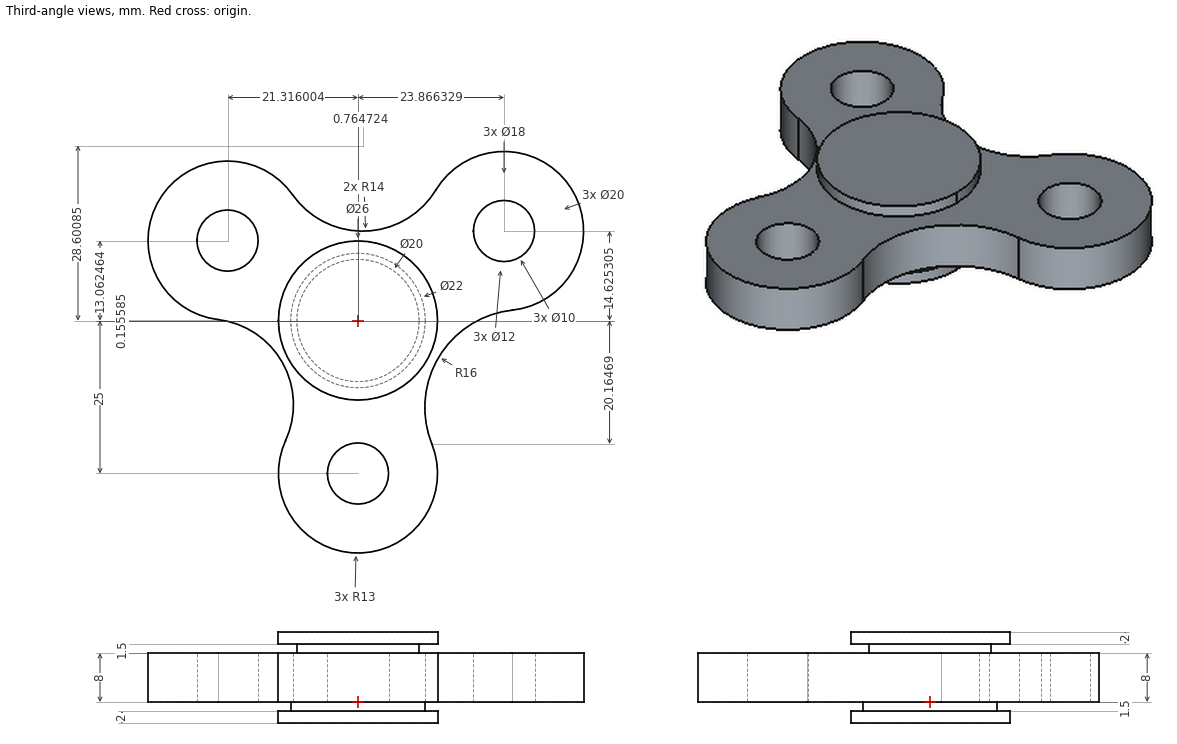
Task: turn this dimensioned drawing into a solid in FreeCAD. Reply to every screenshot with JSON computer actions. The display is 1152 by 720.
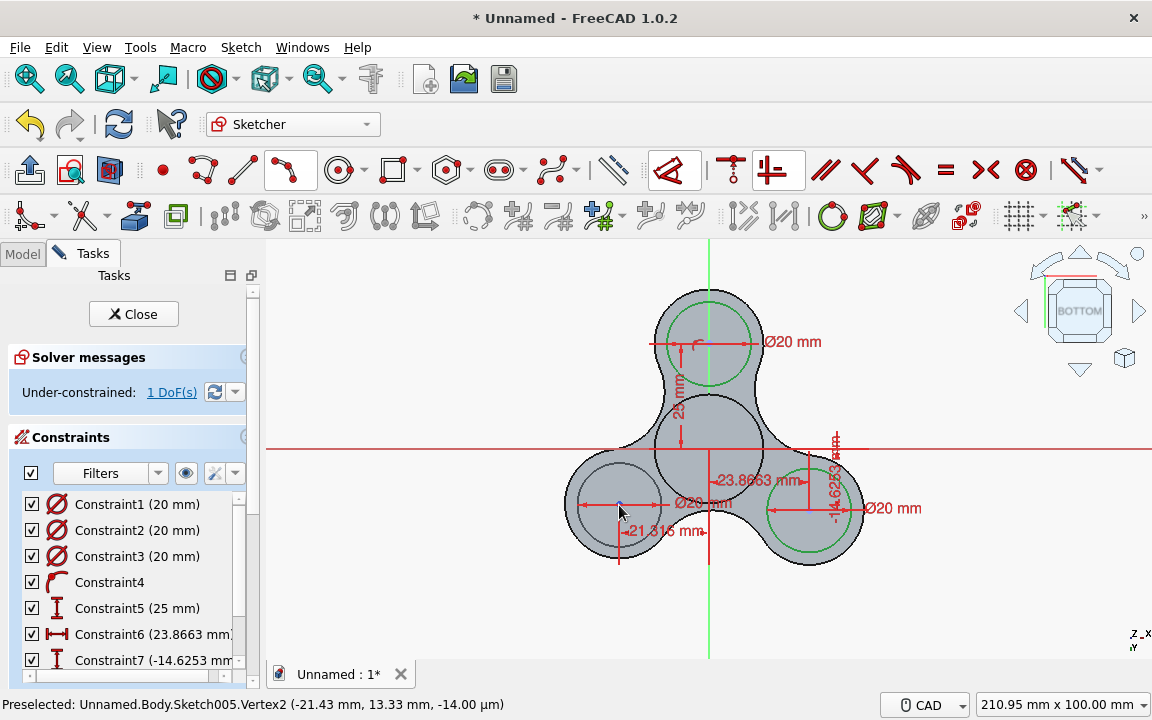
{"action": "left_click", "coordinate": [619, 505]}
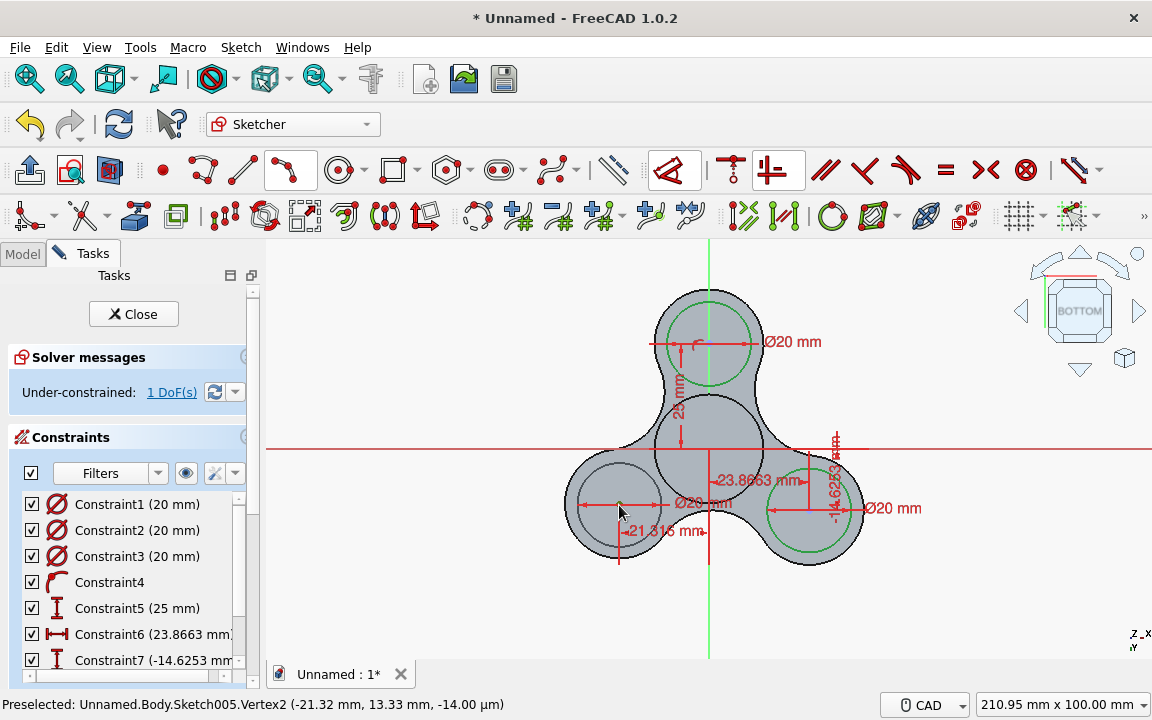
{"action": "key", "text": "i"}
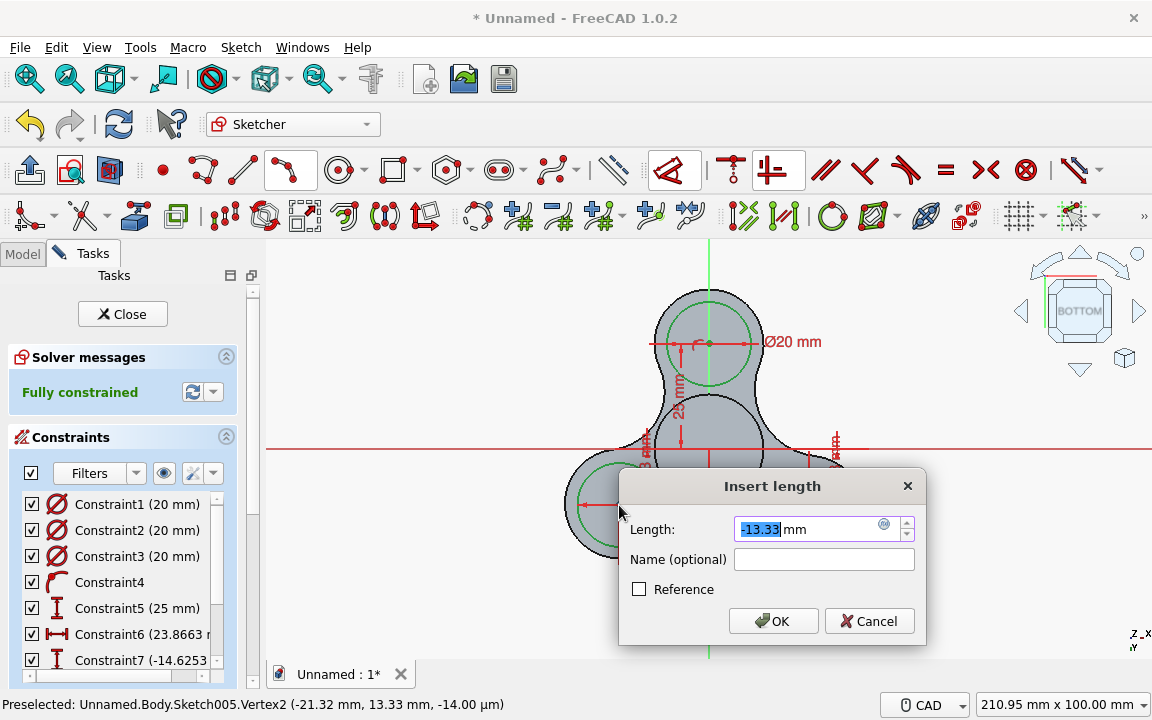
{"action": "type", "text": "-13.062464"}
{"action": "key", "text": "Return"}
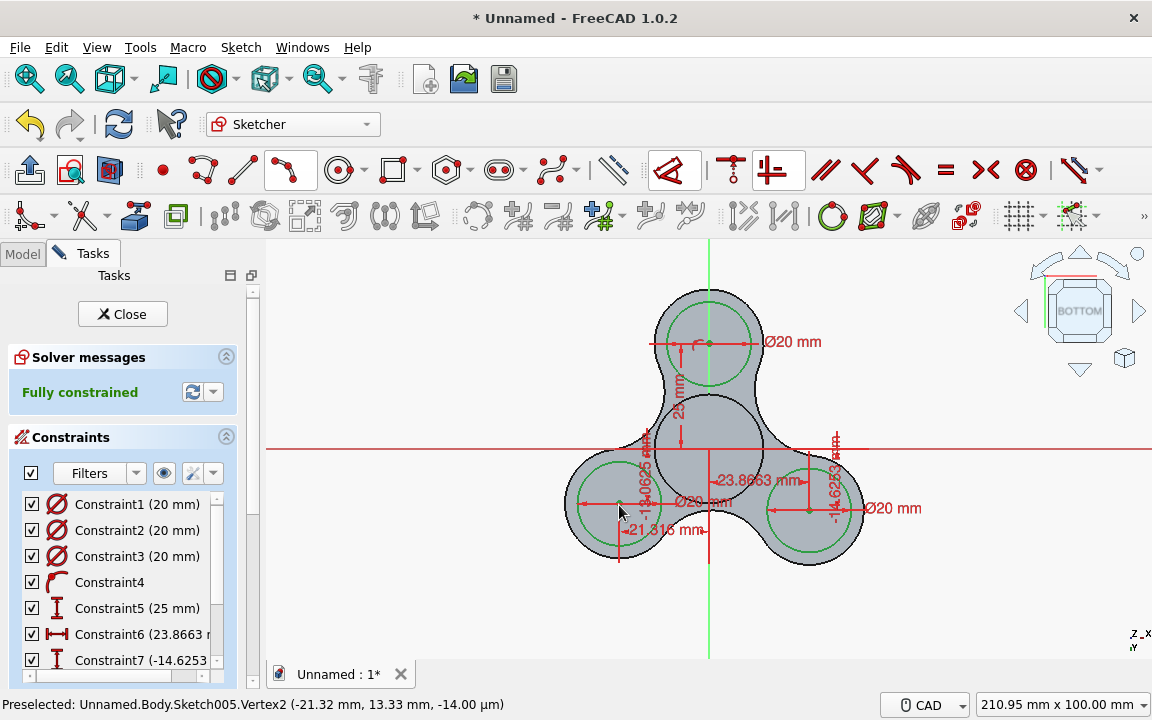
{"action": "left_click", "coordinate": [123, 314]}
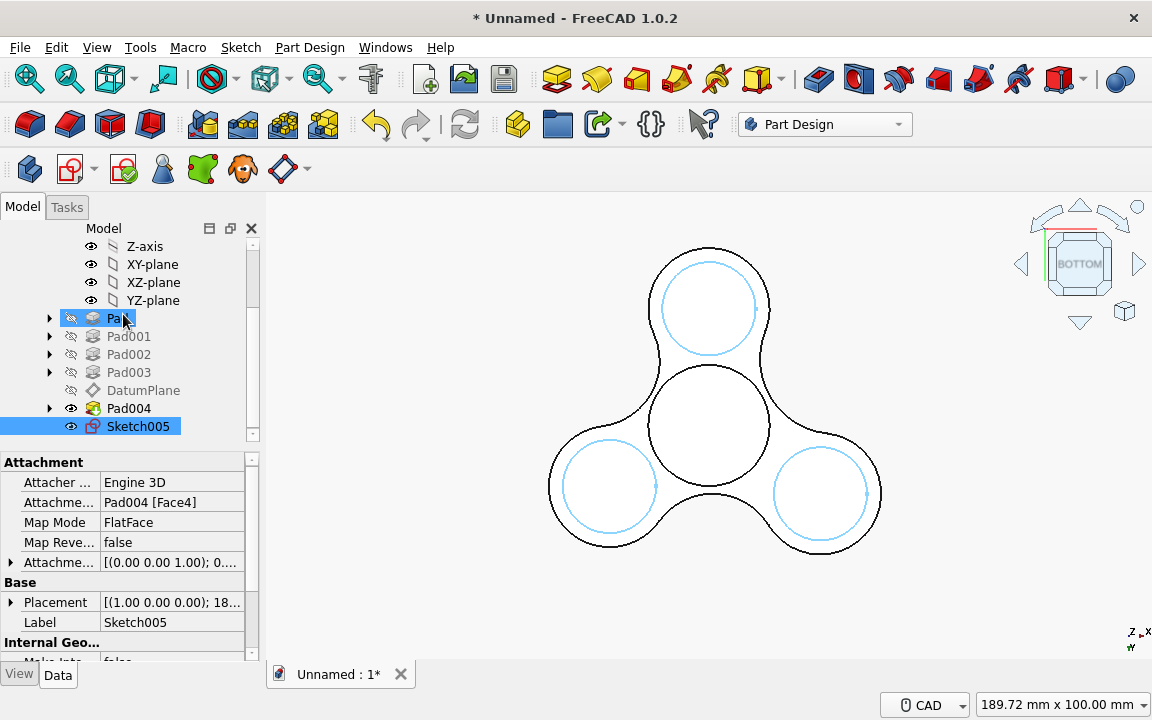
{"action": "left_click", "coordinate": [820, 80]}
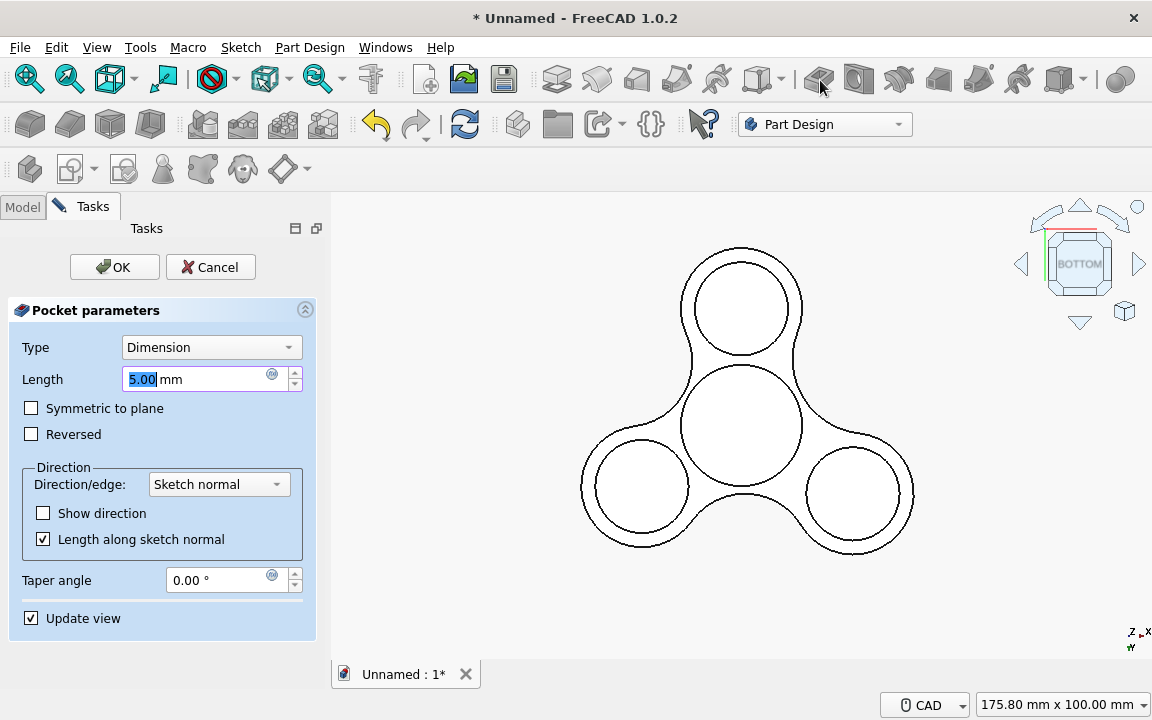
{"action": "type", "text": "8"}
{"action": "key", "text": "Tab"}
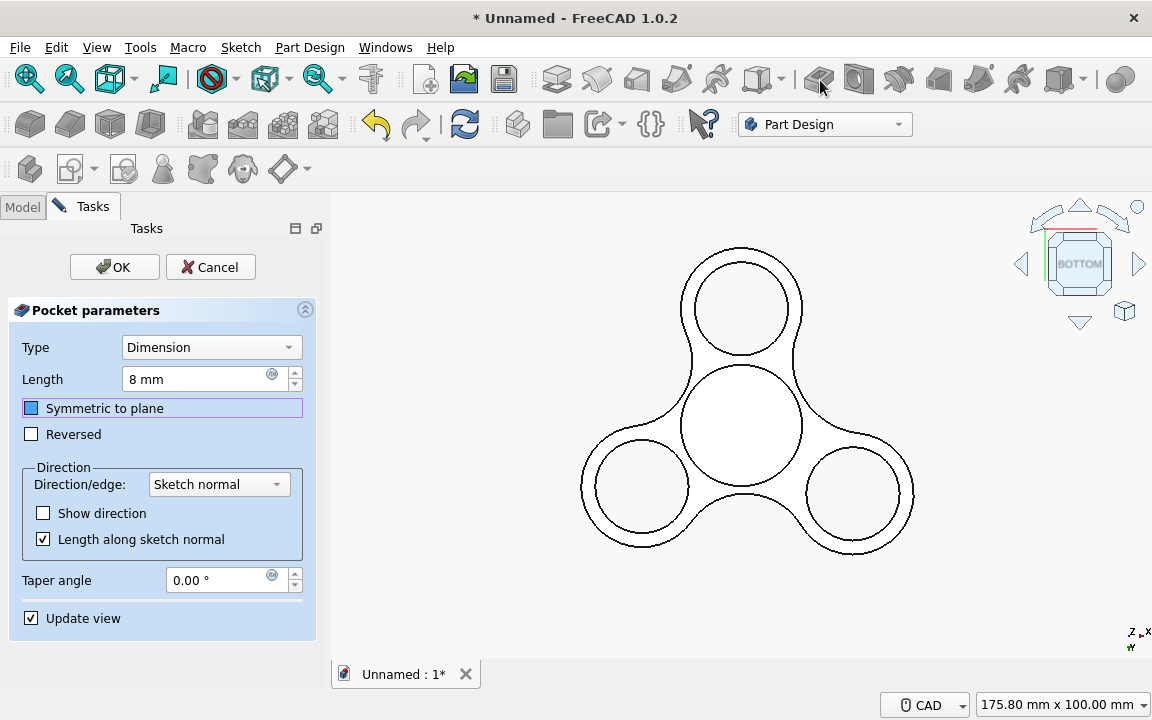
{"action": "left_click", "coordinate": [115, 267]}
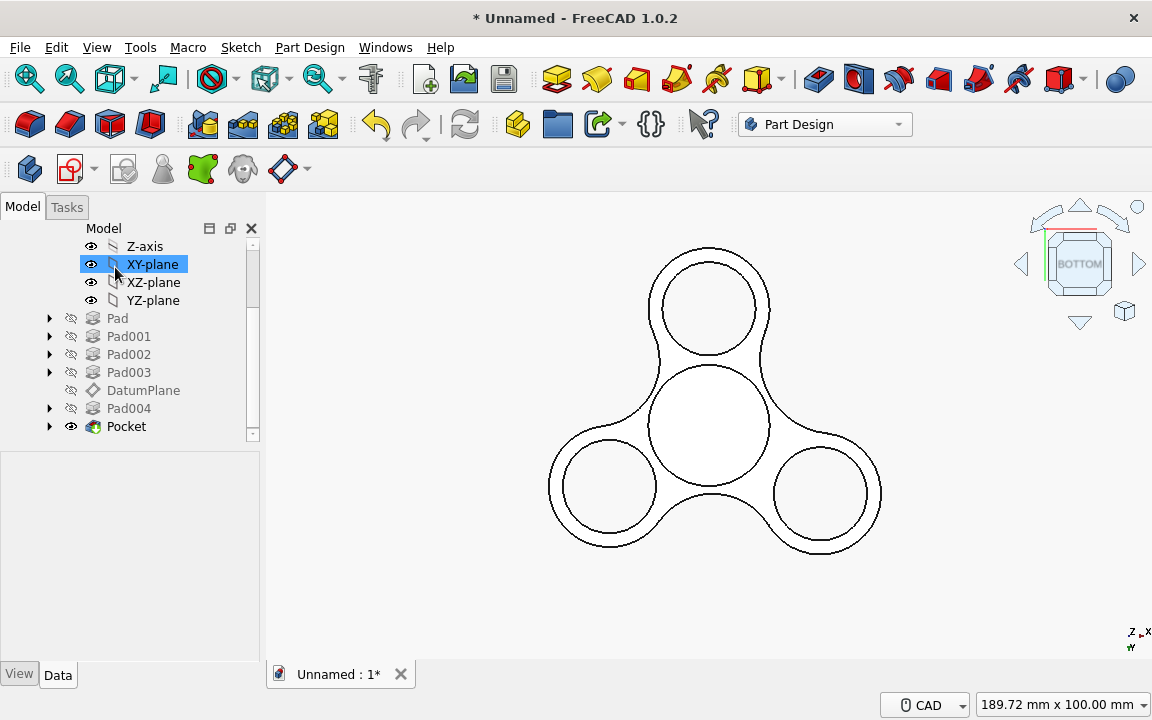
{"action": "left_click", "coordinate": [762, 488]}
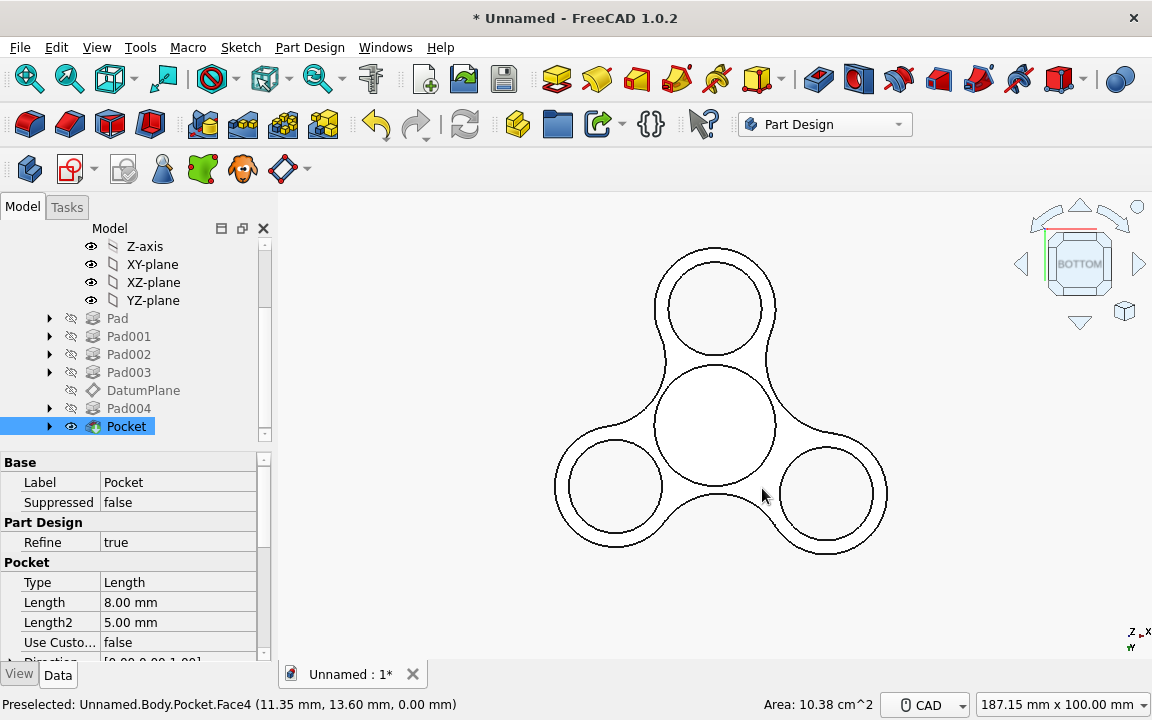
{"action": "left_click", "coordinate": [70, 170]}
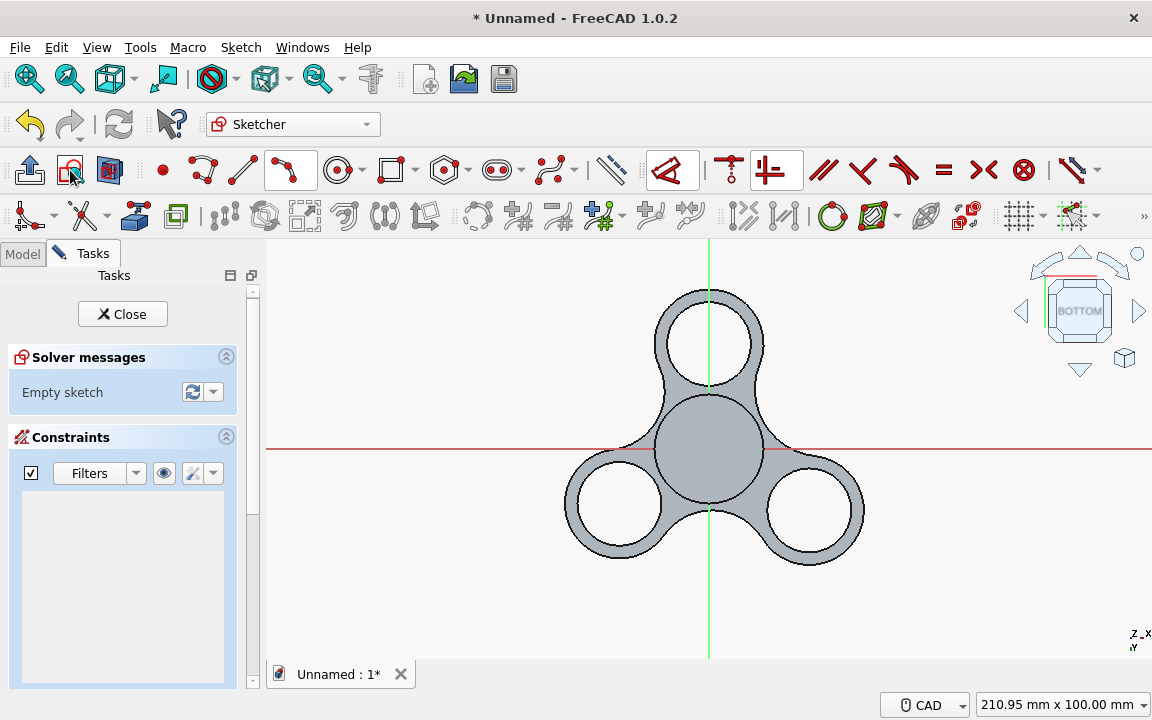
{"action": "left_click", "coordinate": [338, 170]}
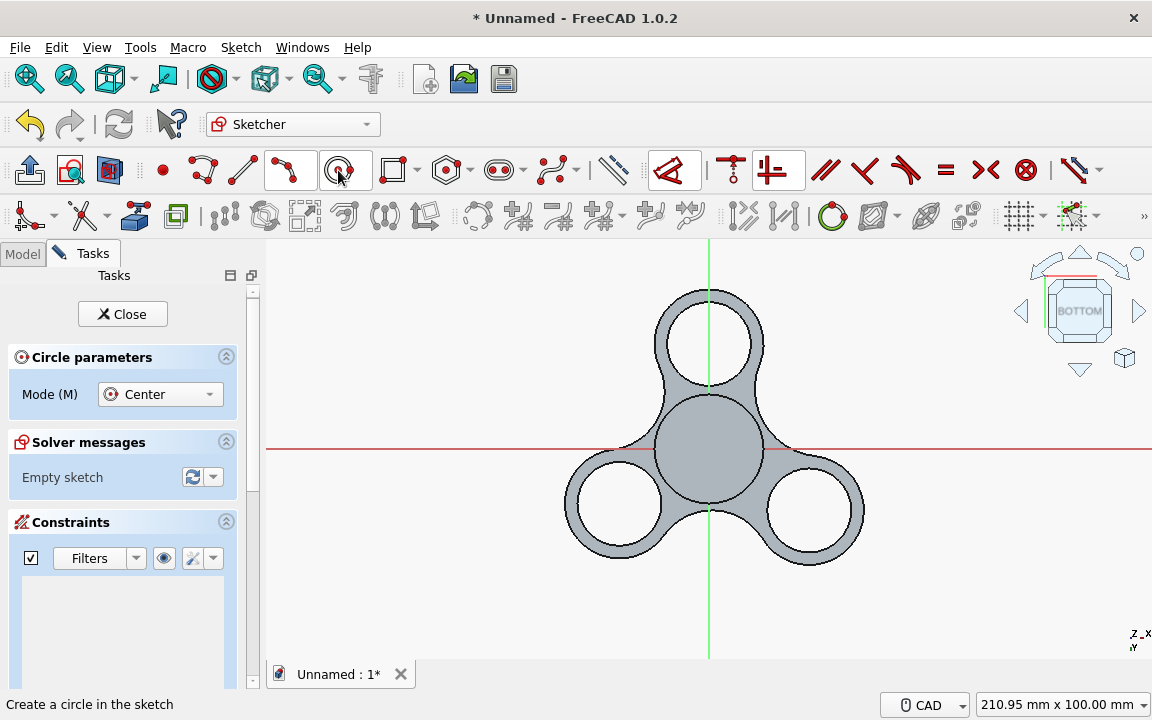
{"action": "left_click", "coordinate": [809, 510]}
{"action": "mouse_move", "coordinate": [839, 481]}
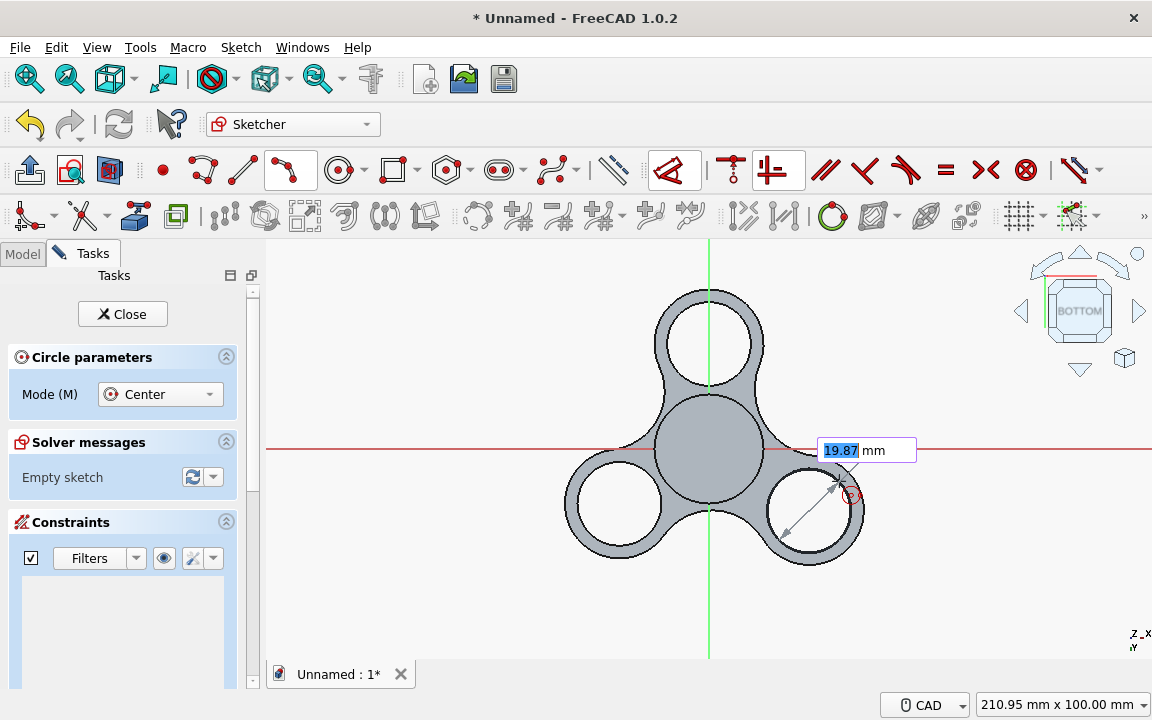
{"action": "type", "text": "20"}
{"action": "key", "text": "Return"}